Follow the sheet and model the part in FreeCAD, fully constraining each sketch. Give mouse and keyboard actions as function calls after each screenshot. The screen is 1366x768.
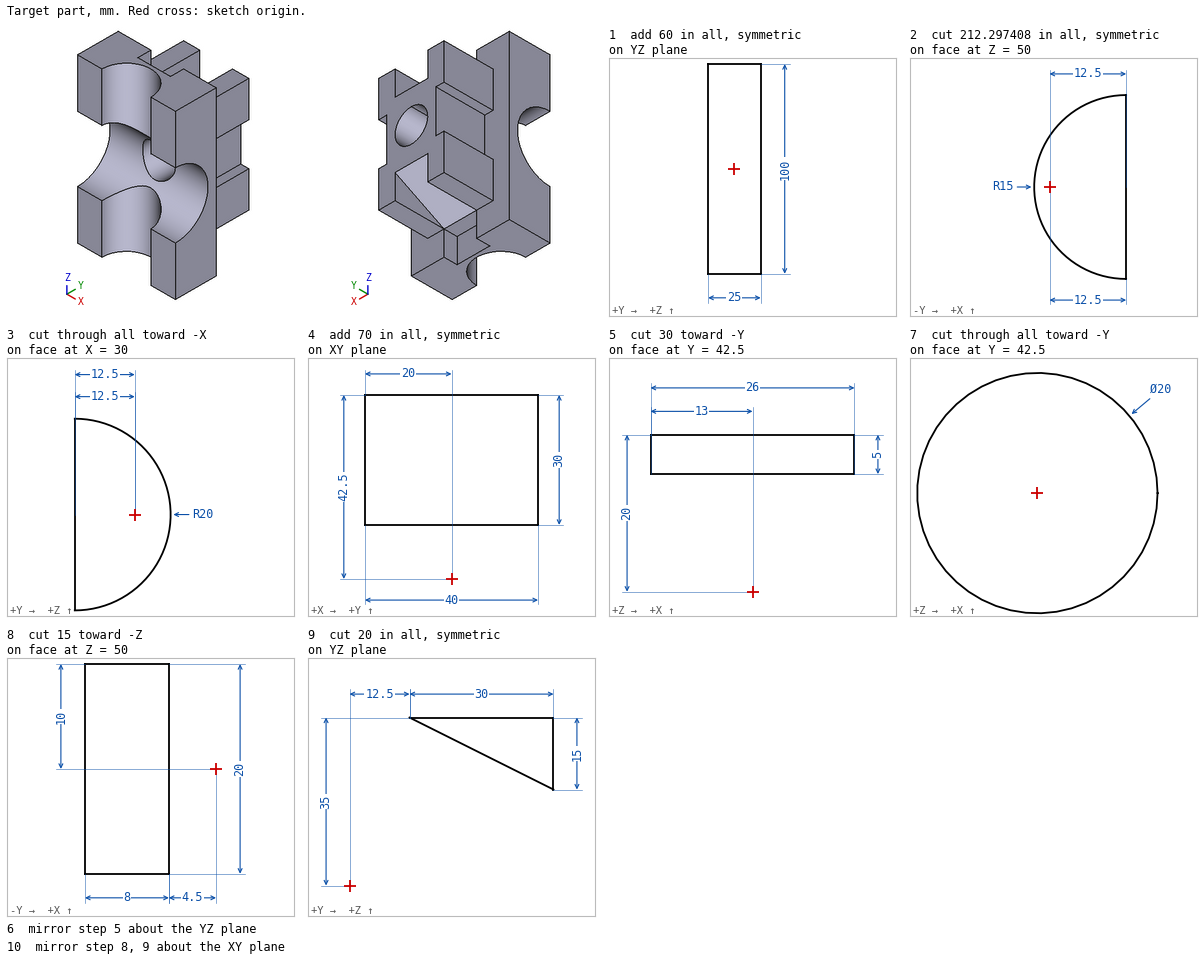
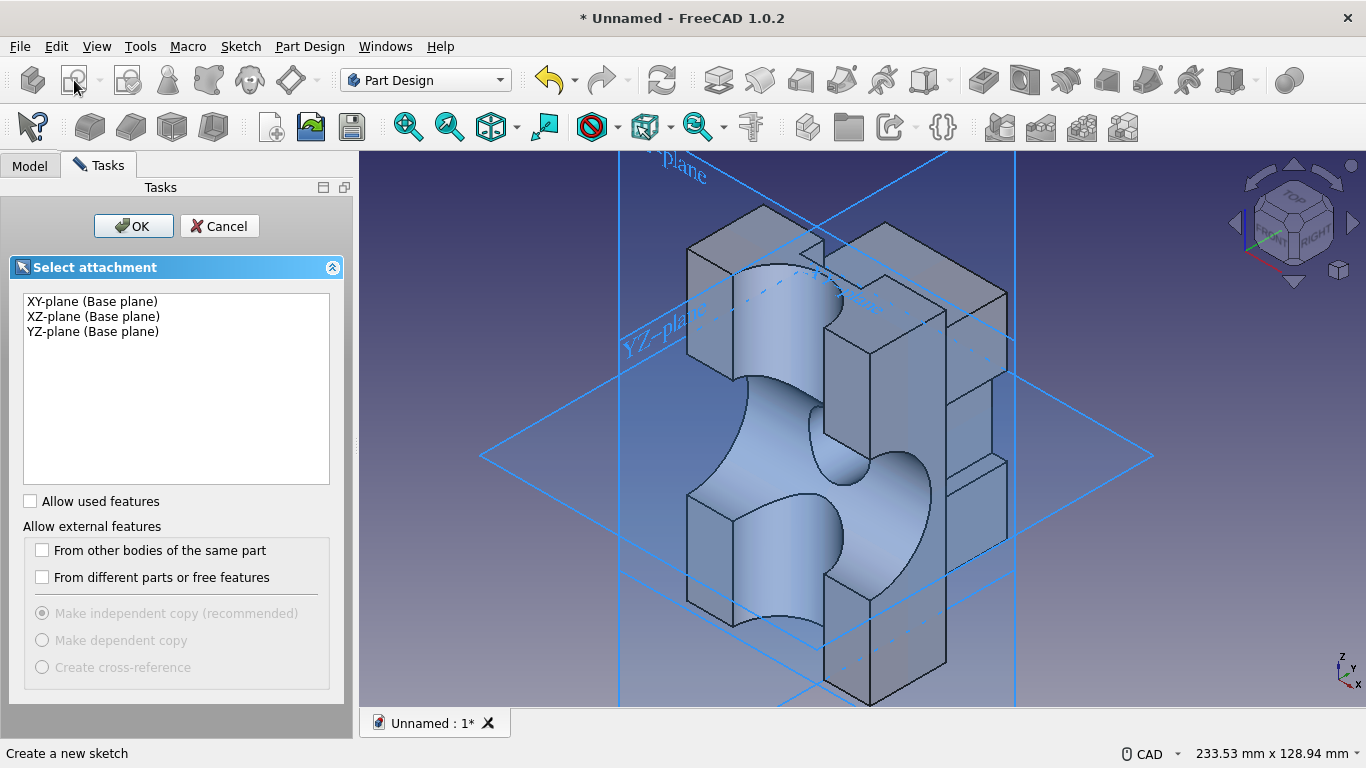
click(84, 332)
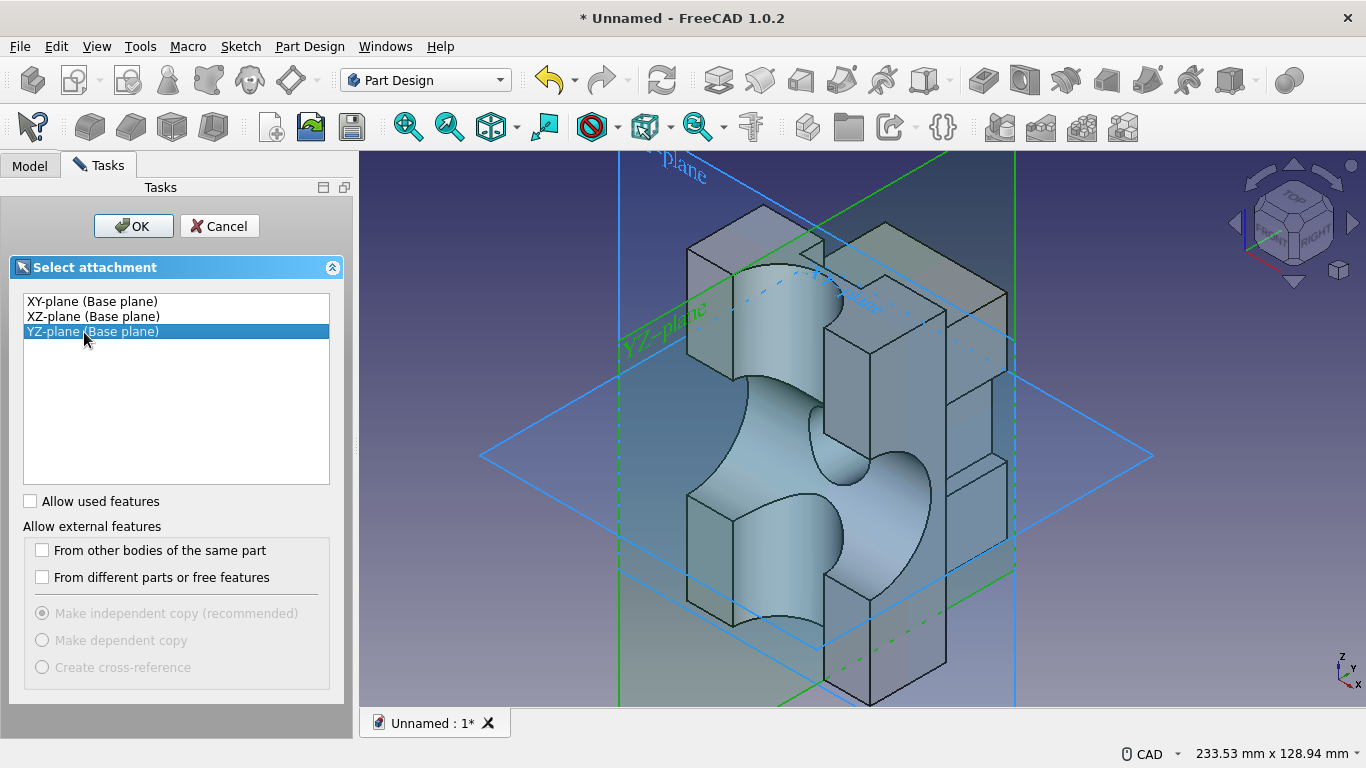
click(134, 226)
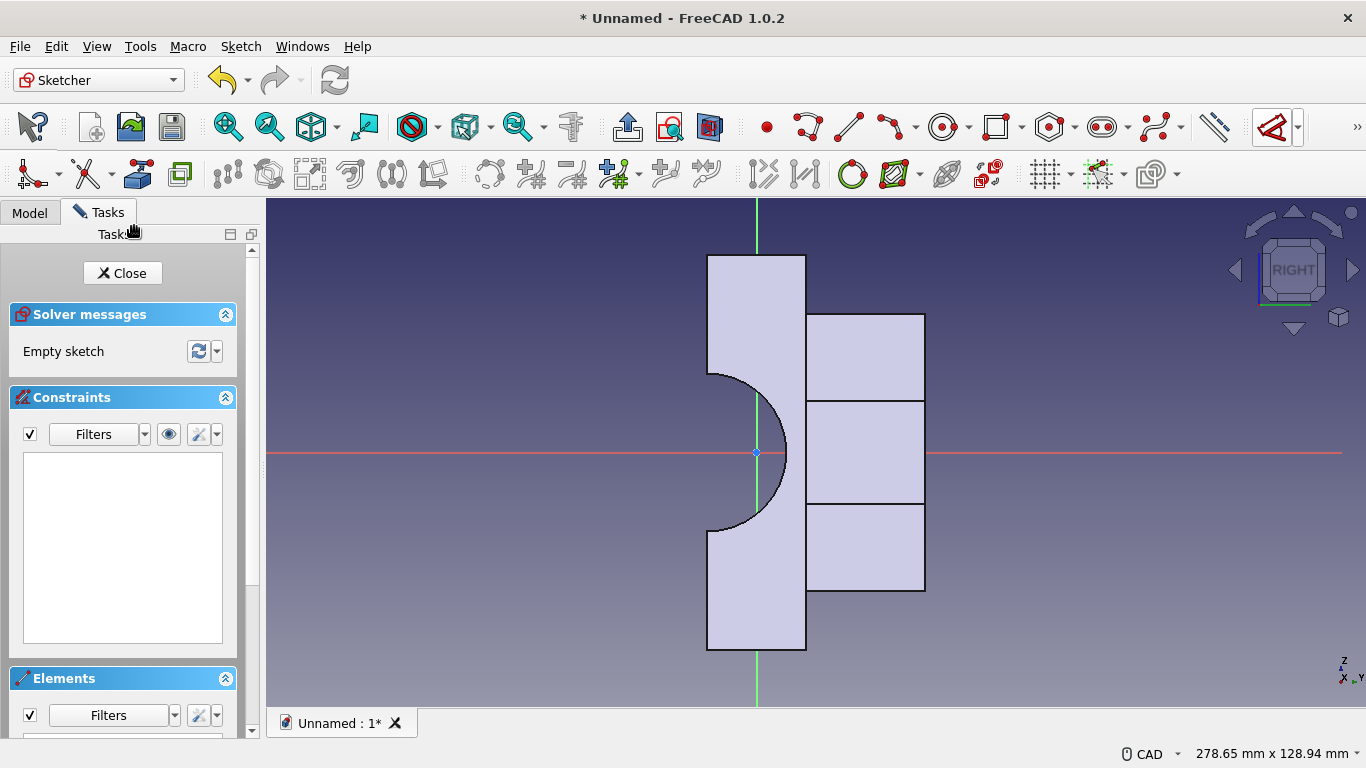
key(q)
key(s)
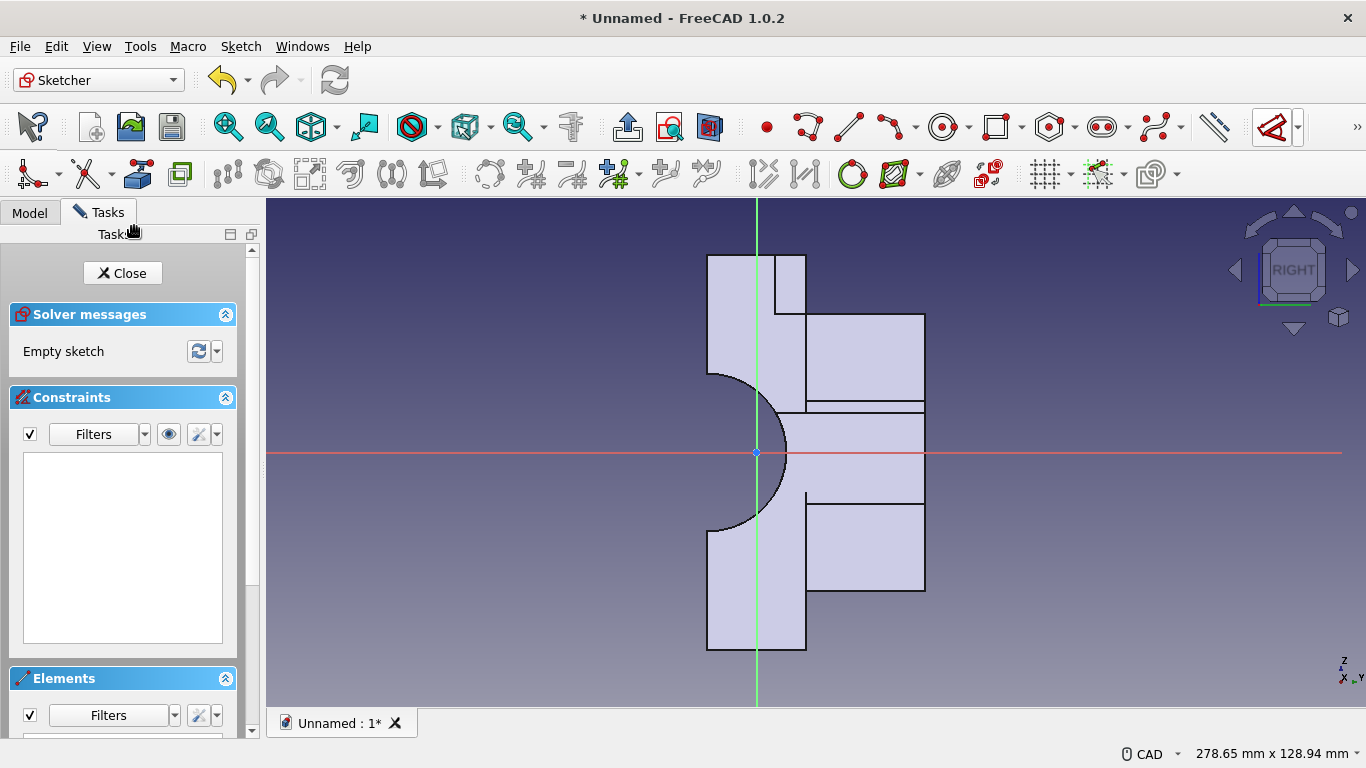
scroll(917, 327, up, 4)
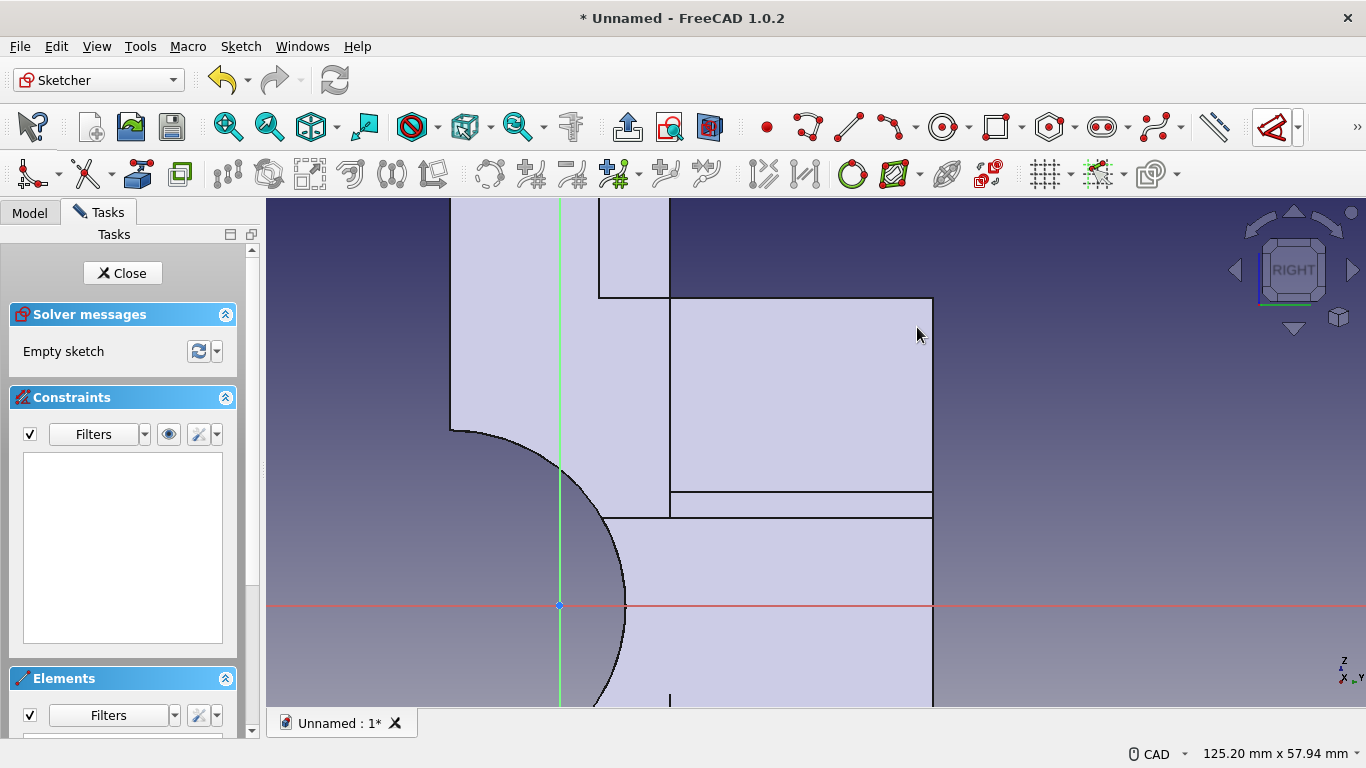
click(808, 128)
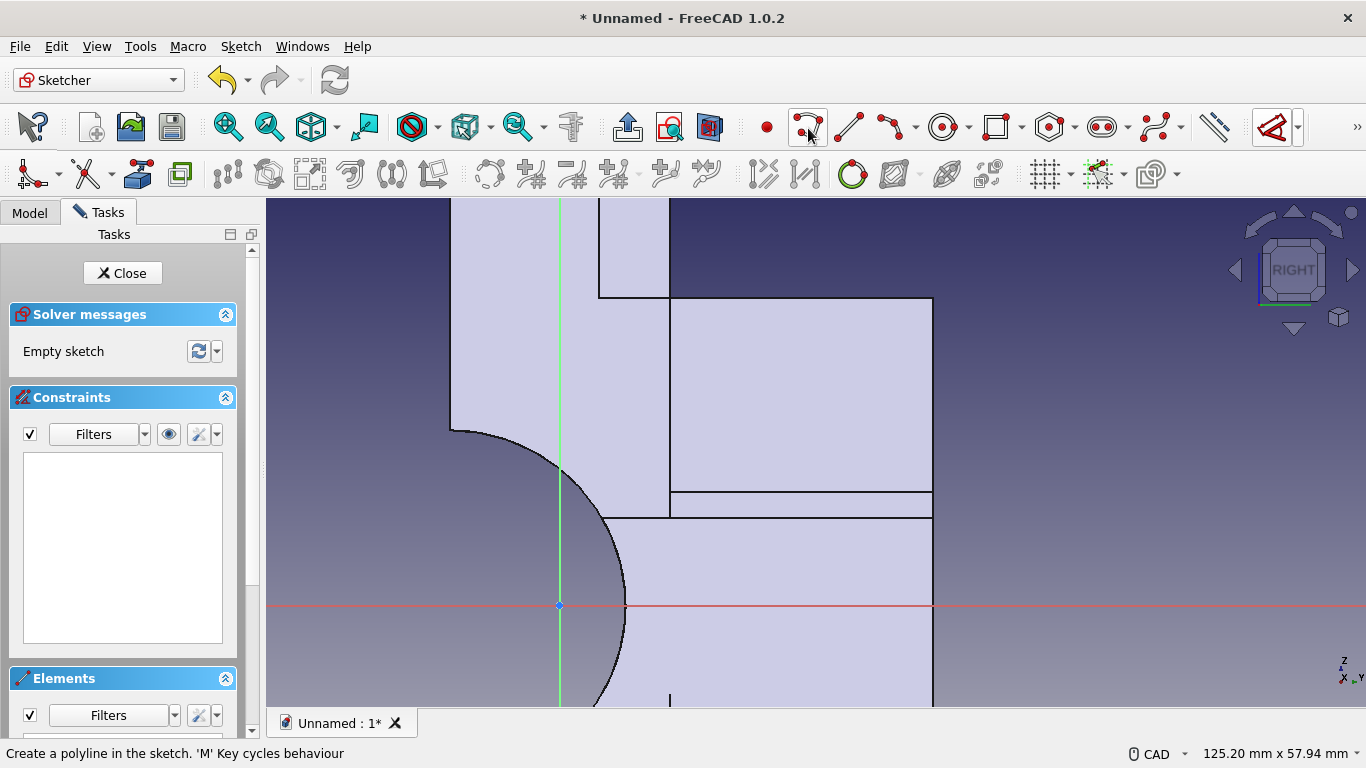
click(670, 298)
click(933, 430)
click(933, 298)
click(670, 299)
key(Escape)
key(Escape)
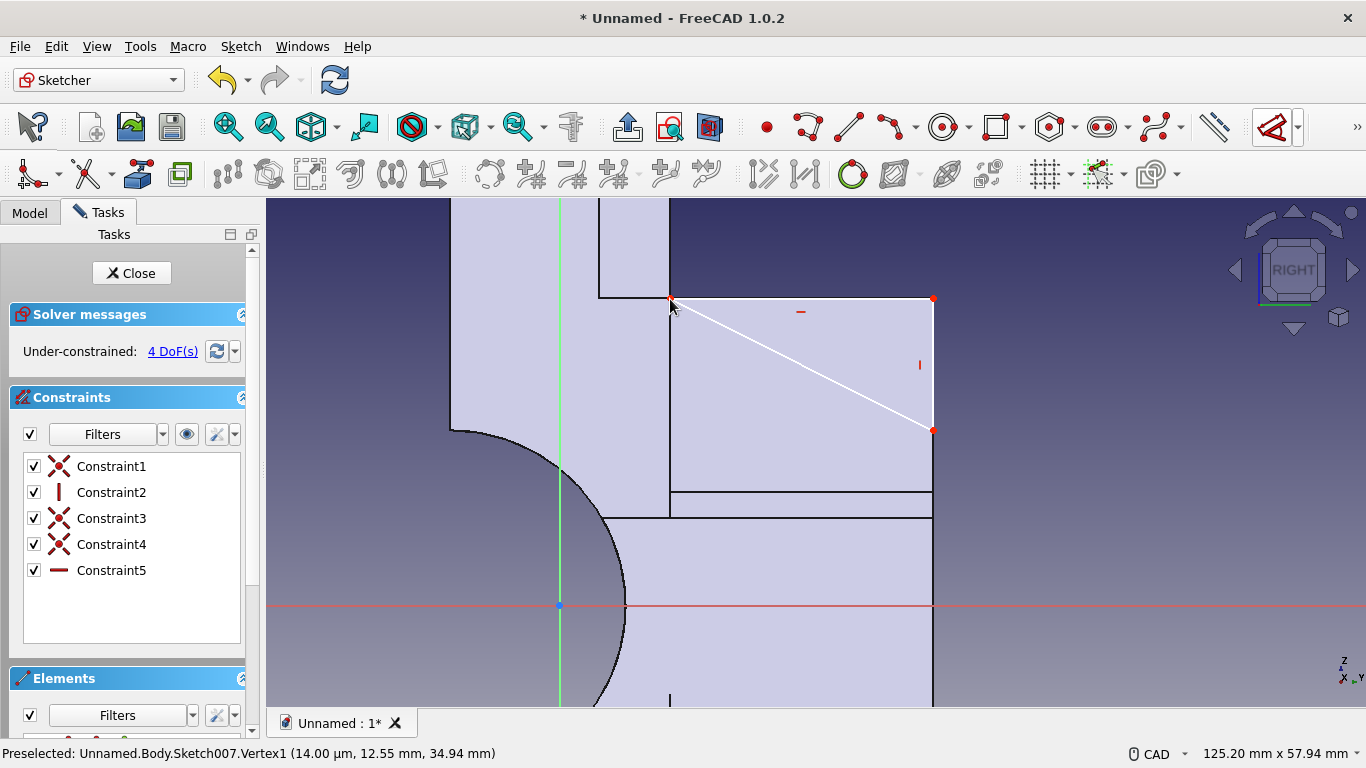
click(933, 391)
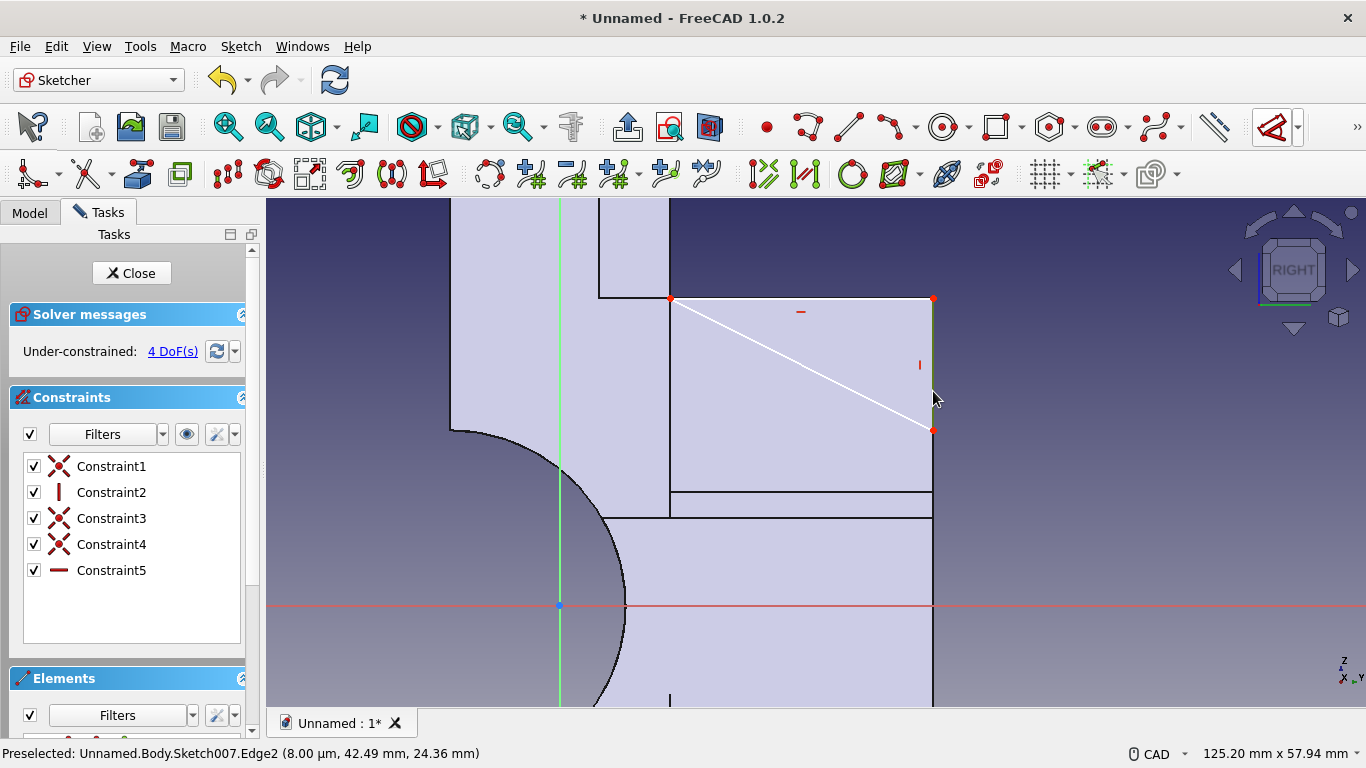
click(1298, 128)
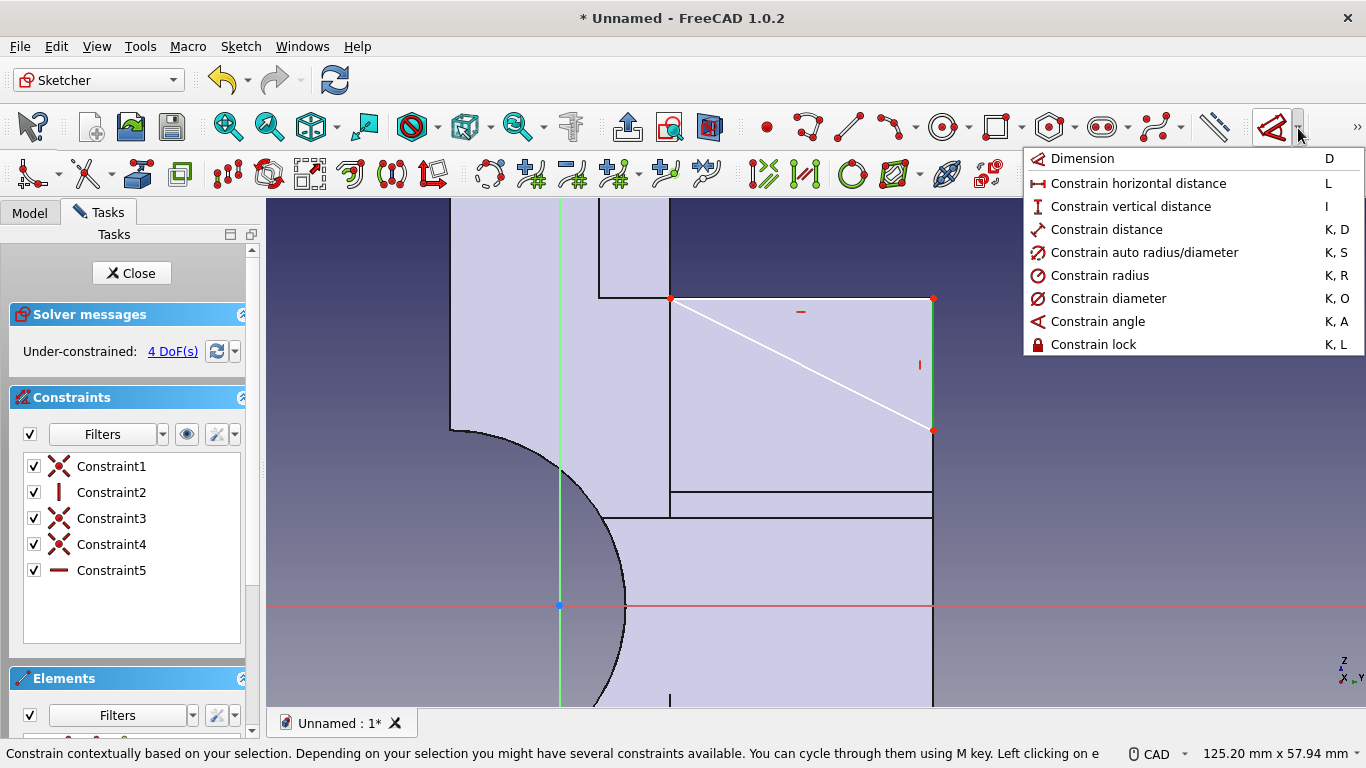
click(1194, 206)